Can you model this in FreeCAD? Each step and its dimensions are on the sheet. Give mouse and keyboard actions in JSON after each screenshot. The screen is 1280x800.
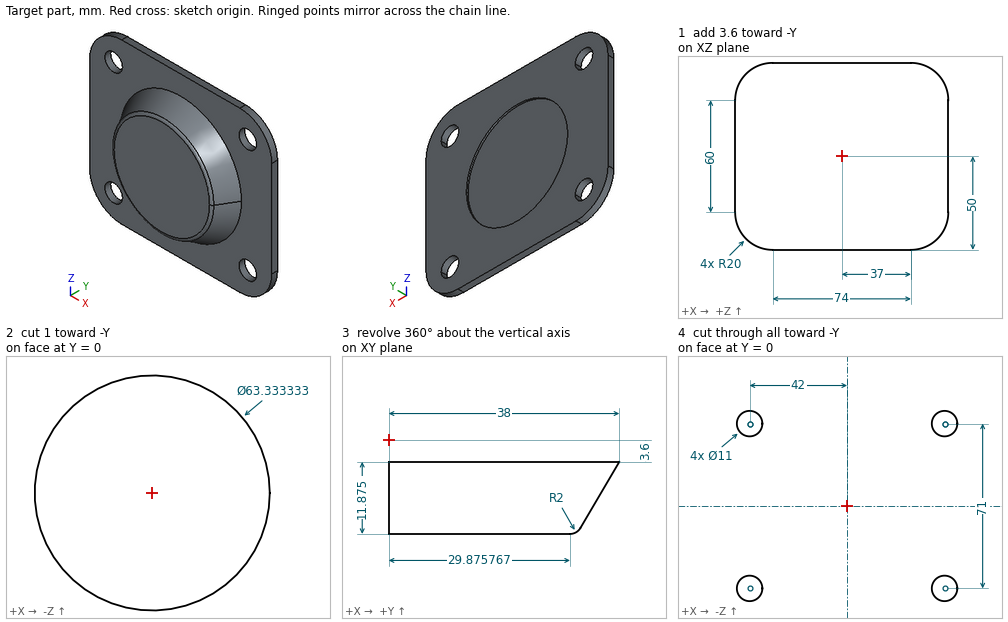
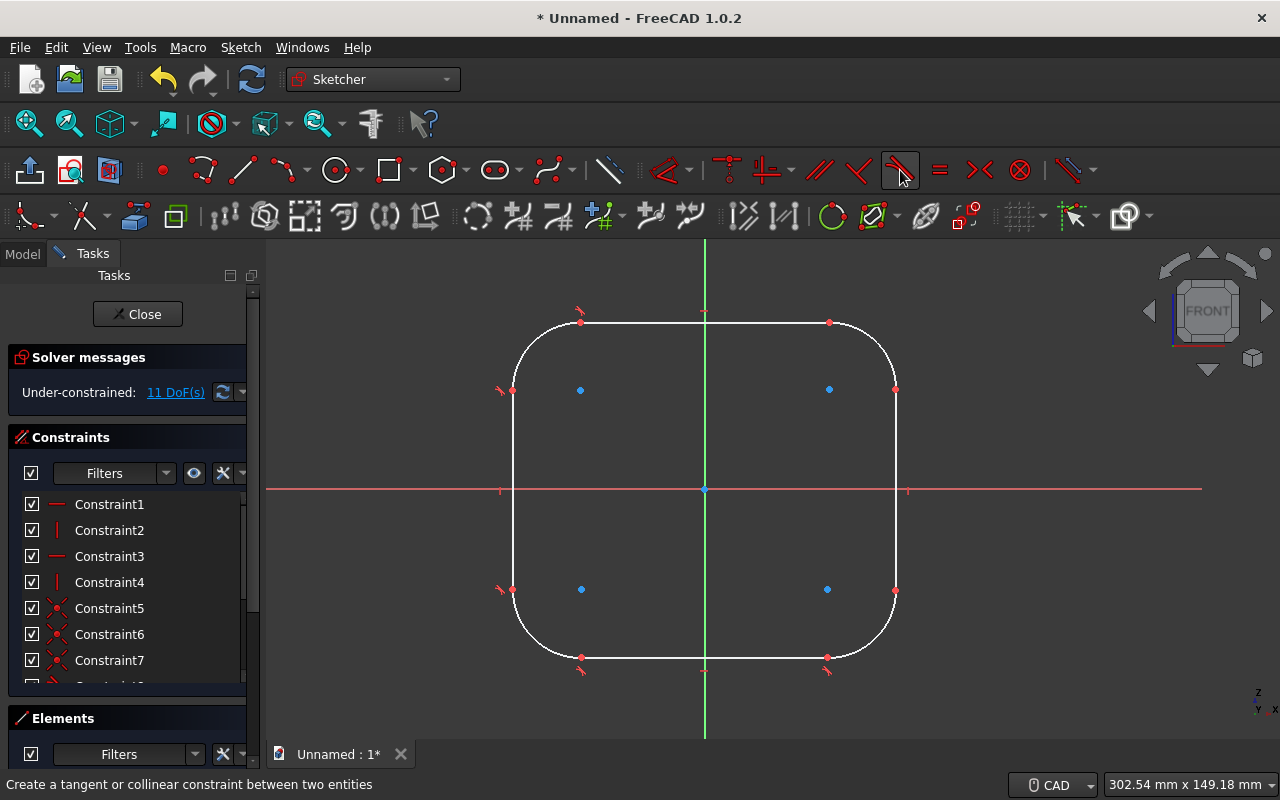
{"action": "left_click", "coordinate": [655, 323]}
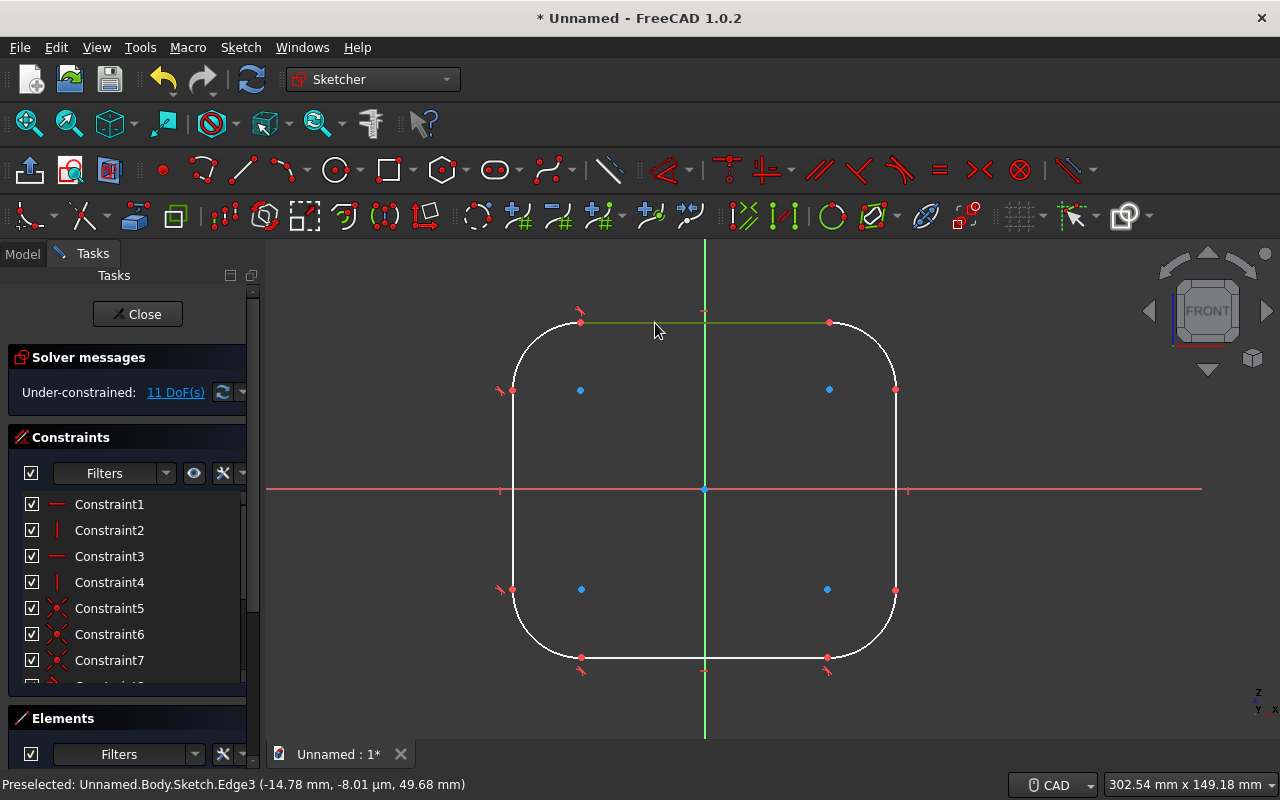
{"action": "left_click", "coordinate": [889, 359]}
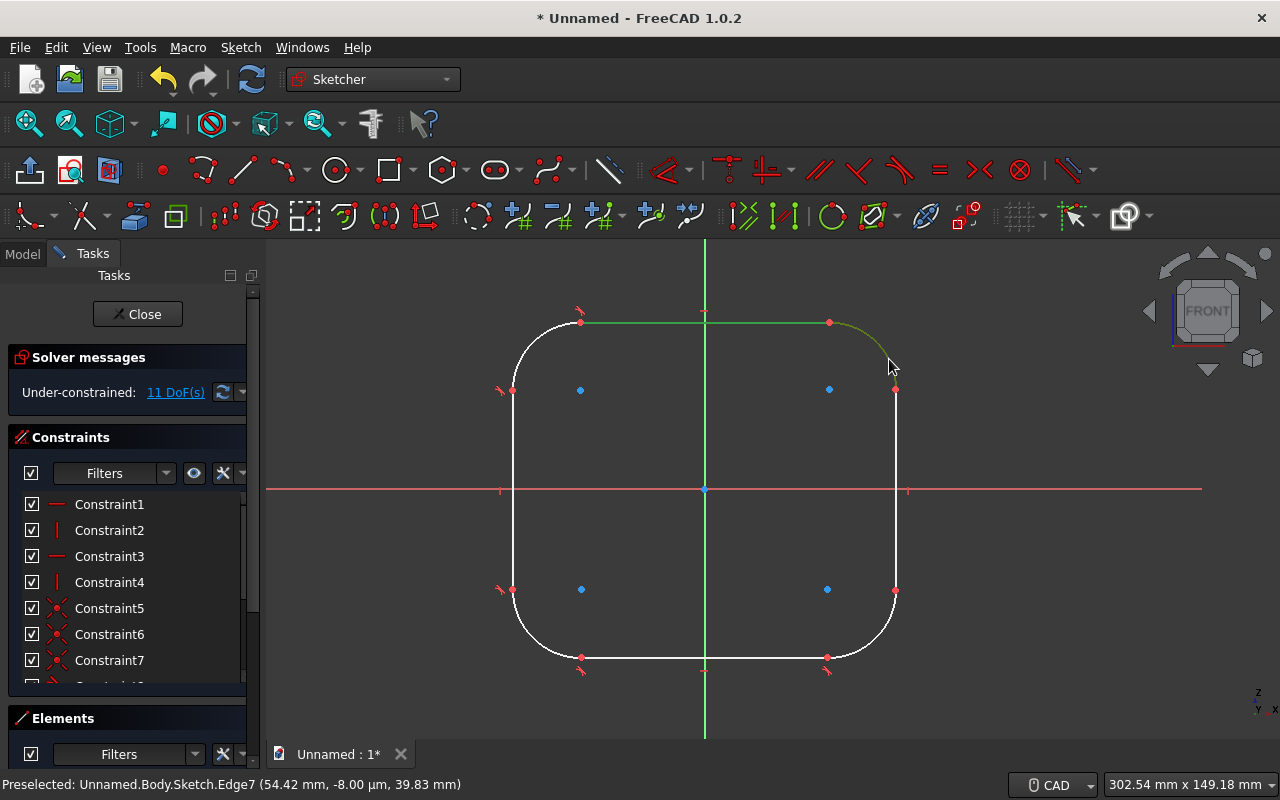
{"action": "left_click", "coordinate": [900, 170]}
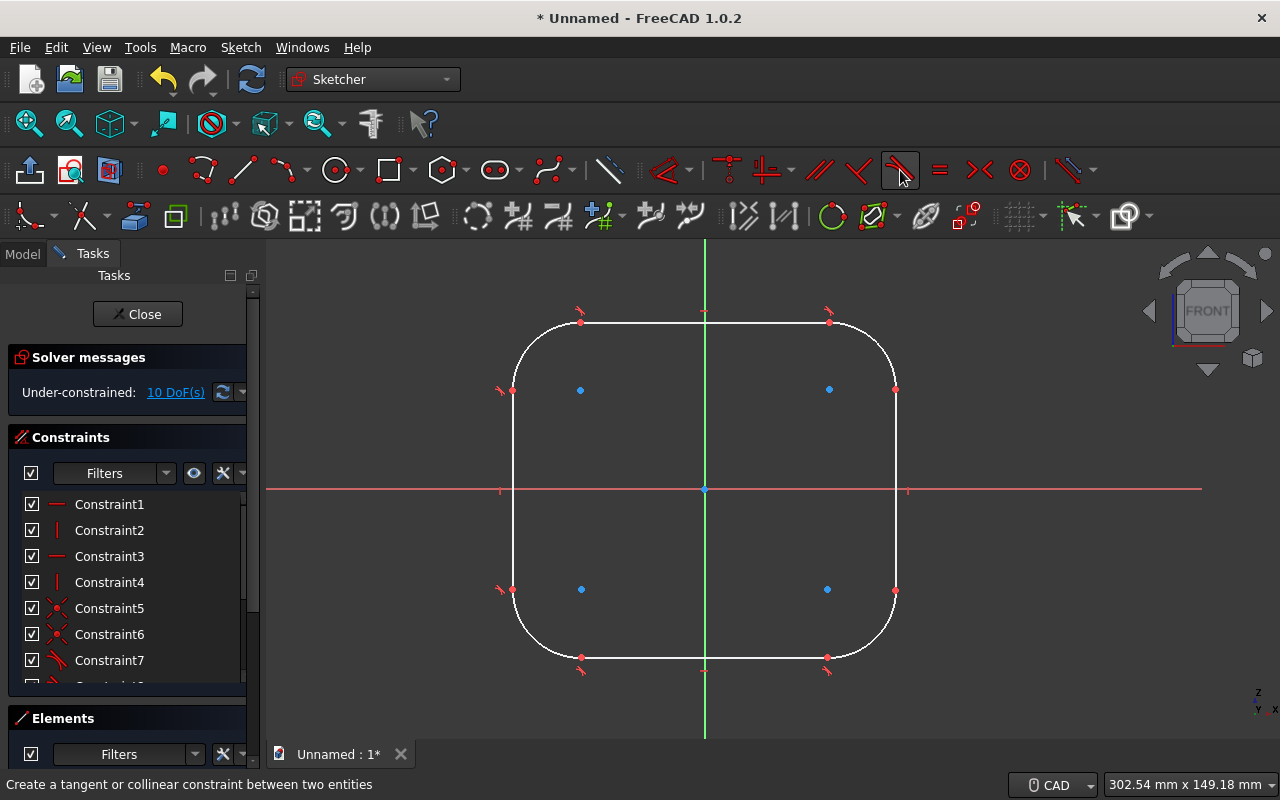
{"action": "left_click", "coordinate": [896, 450]}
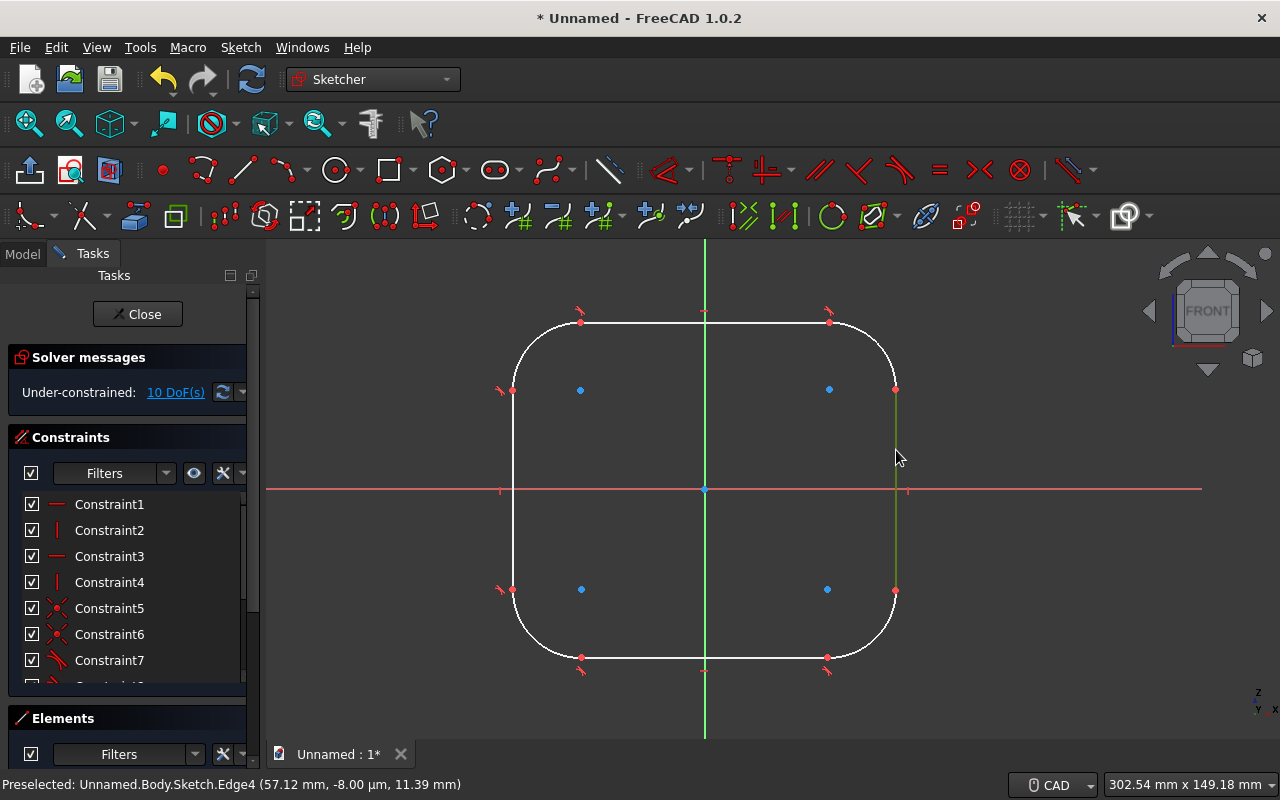
{"action": "left_click", "coordinate": [889, 359]}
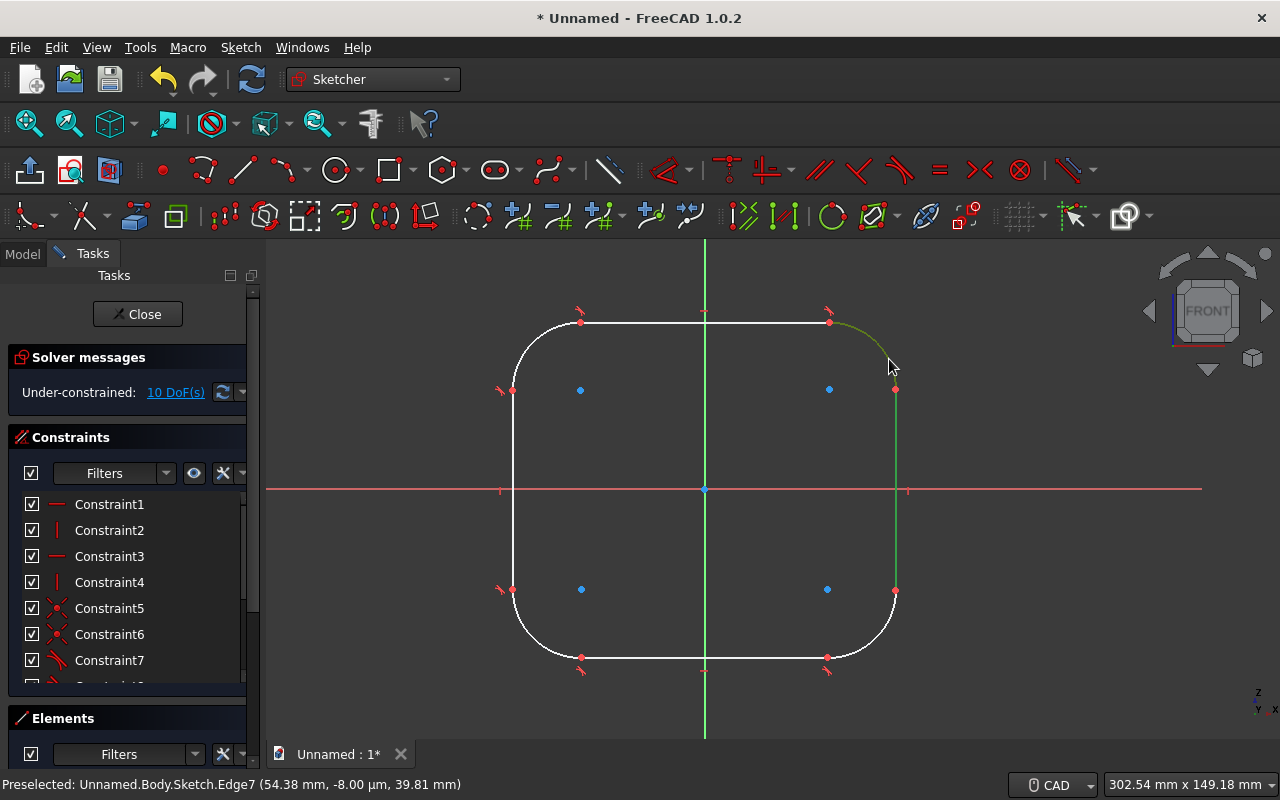
{"action": "left_click", "coordinate": [900, 170]}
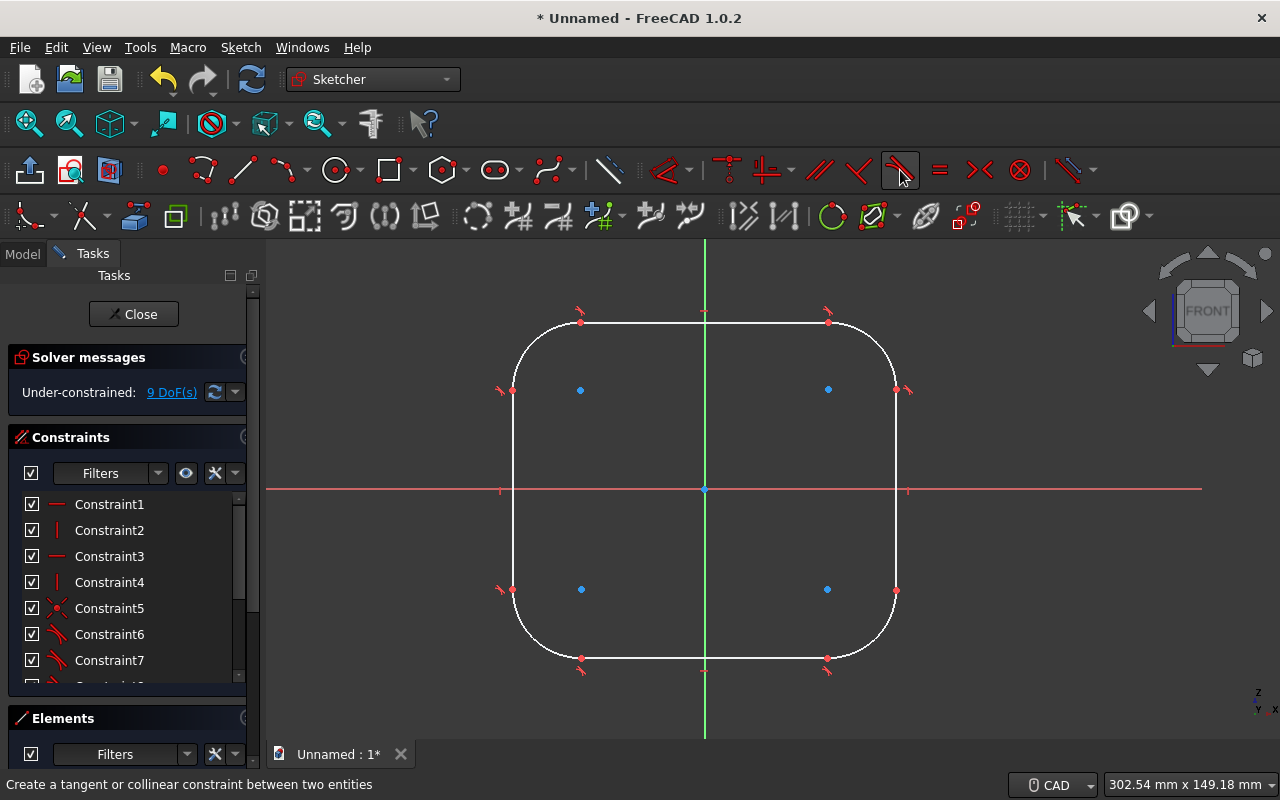
{"action": "left_click", "coordinate": [896, 450]}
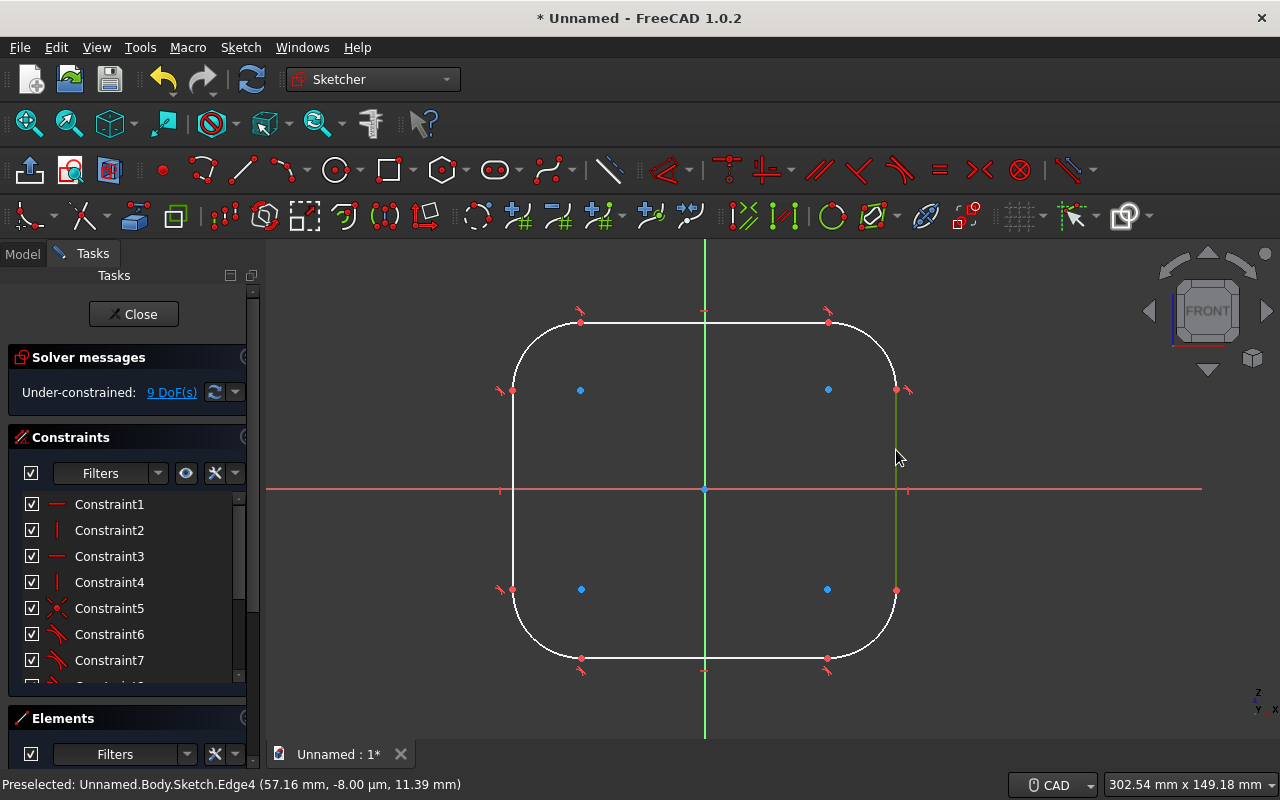
{"action": "left_click", "coordinate": [858, 651]}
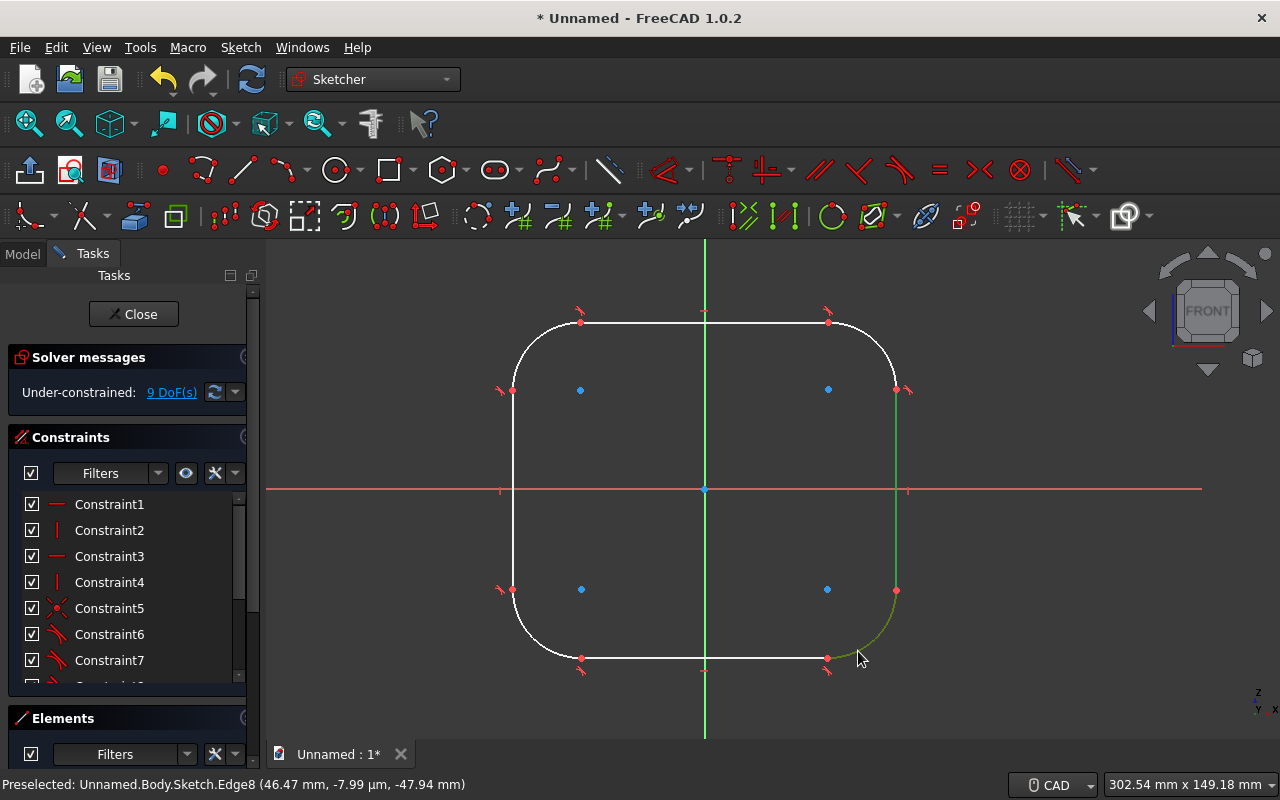
{"action": "left_click", "coordinate": [900, 170]}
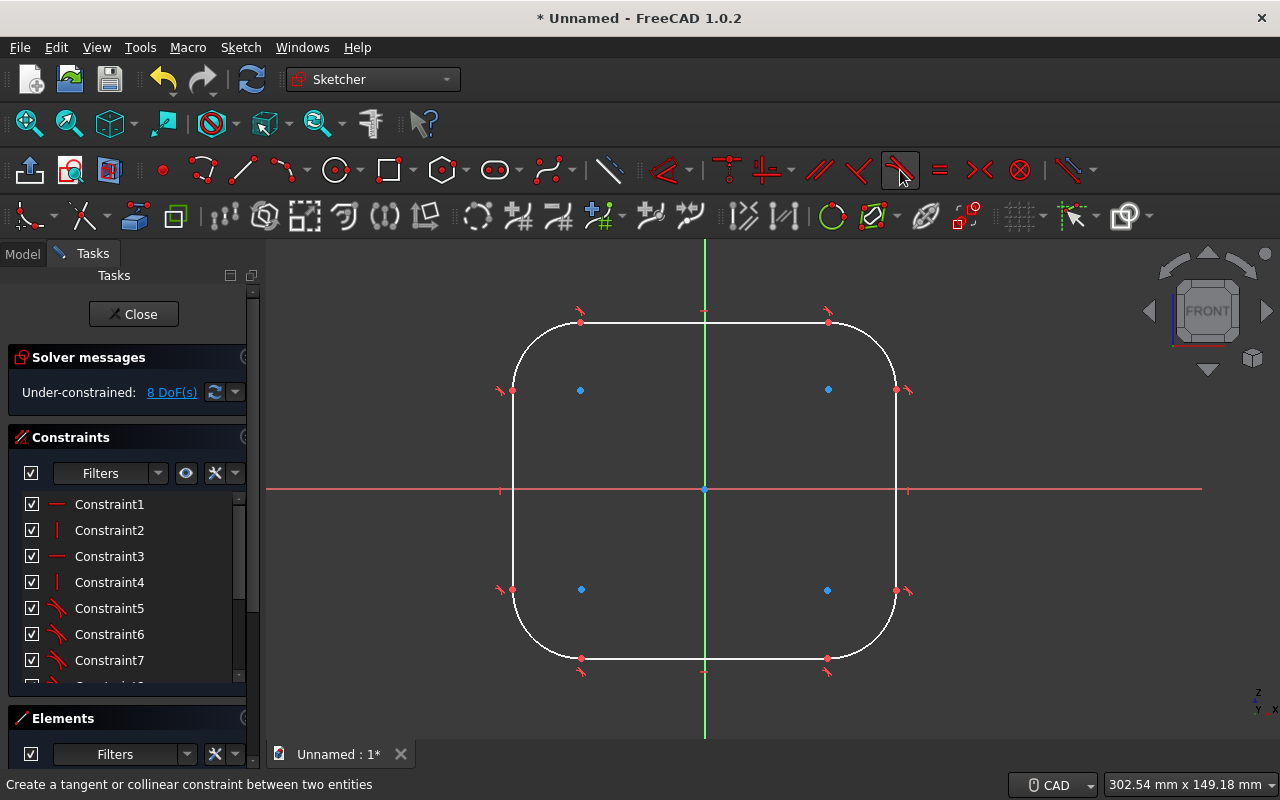
{"action": "left_click", "coordinate": [520, 621]}